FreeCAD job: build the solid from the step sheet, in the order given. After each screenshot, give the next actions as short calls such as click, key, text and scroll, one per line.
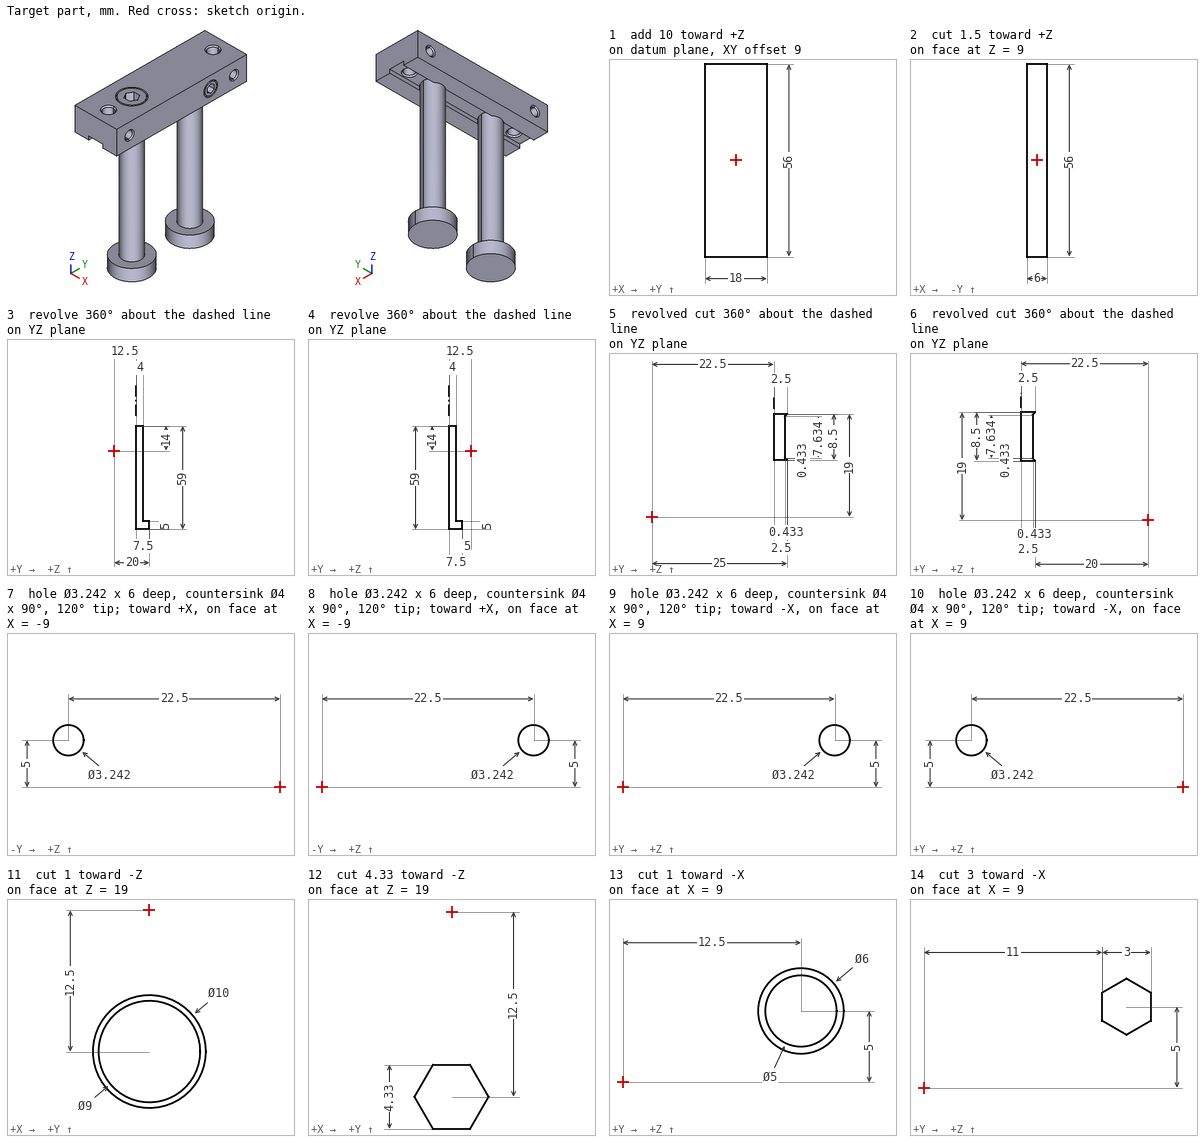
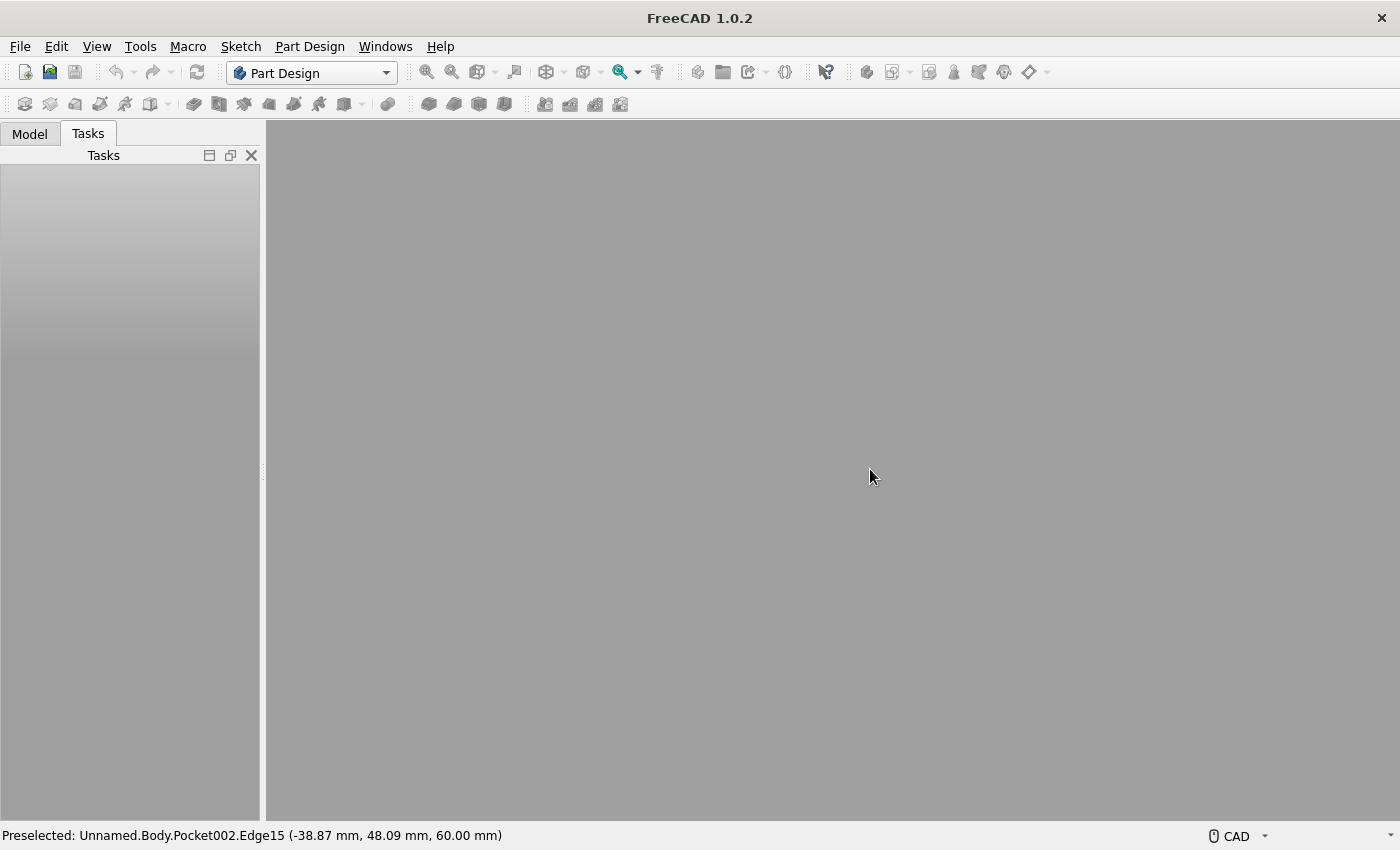
click(25, 72)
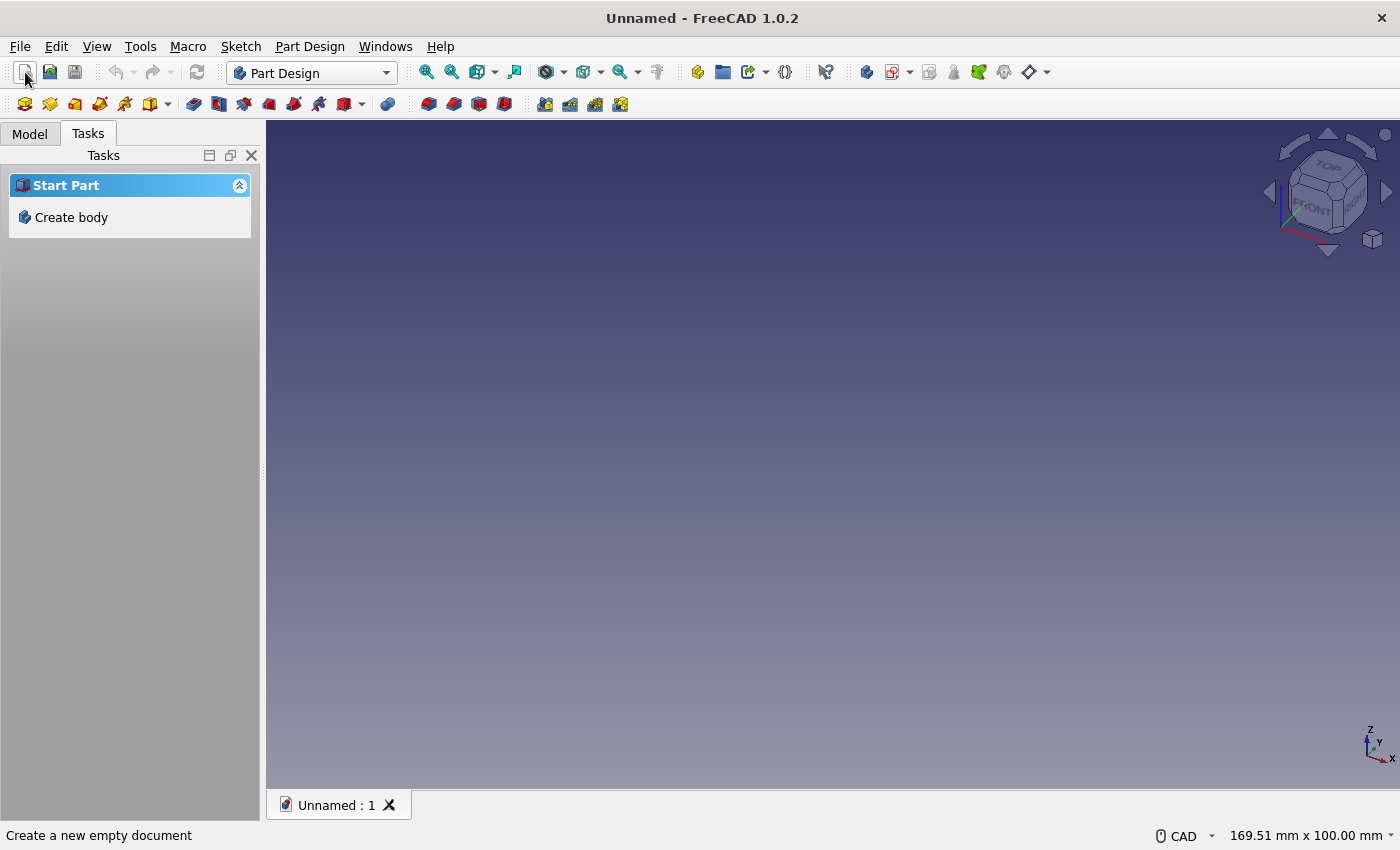
click(867, 72)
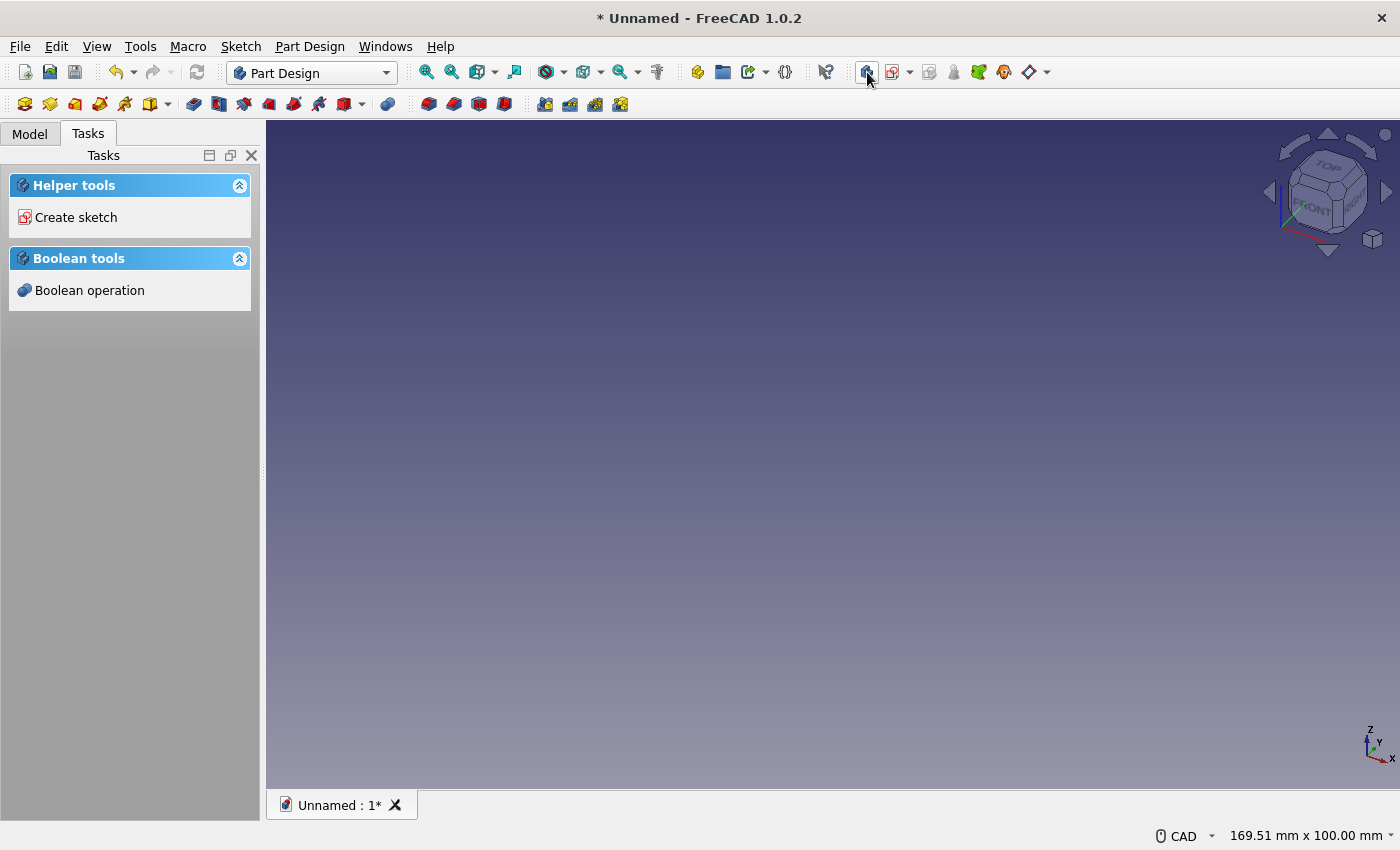
click(30, 134)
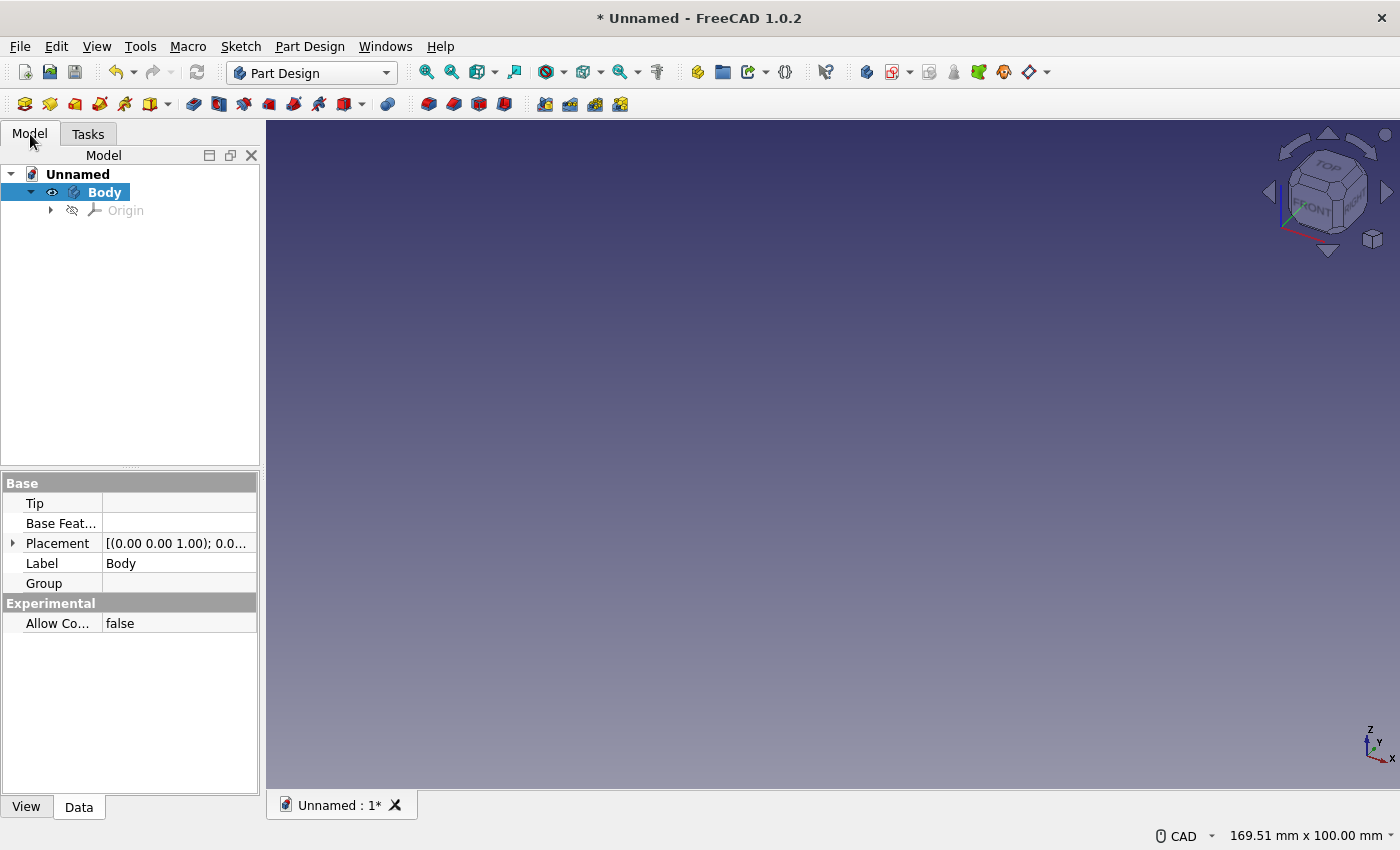
click(51, 210)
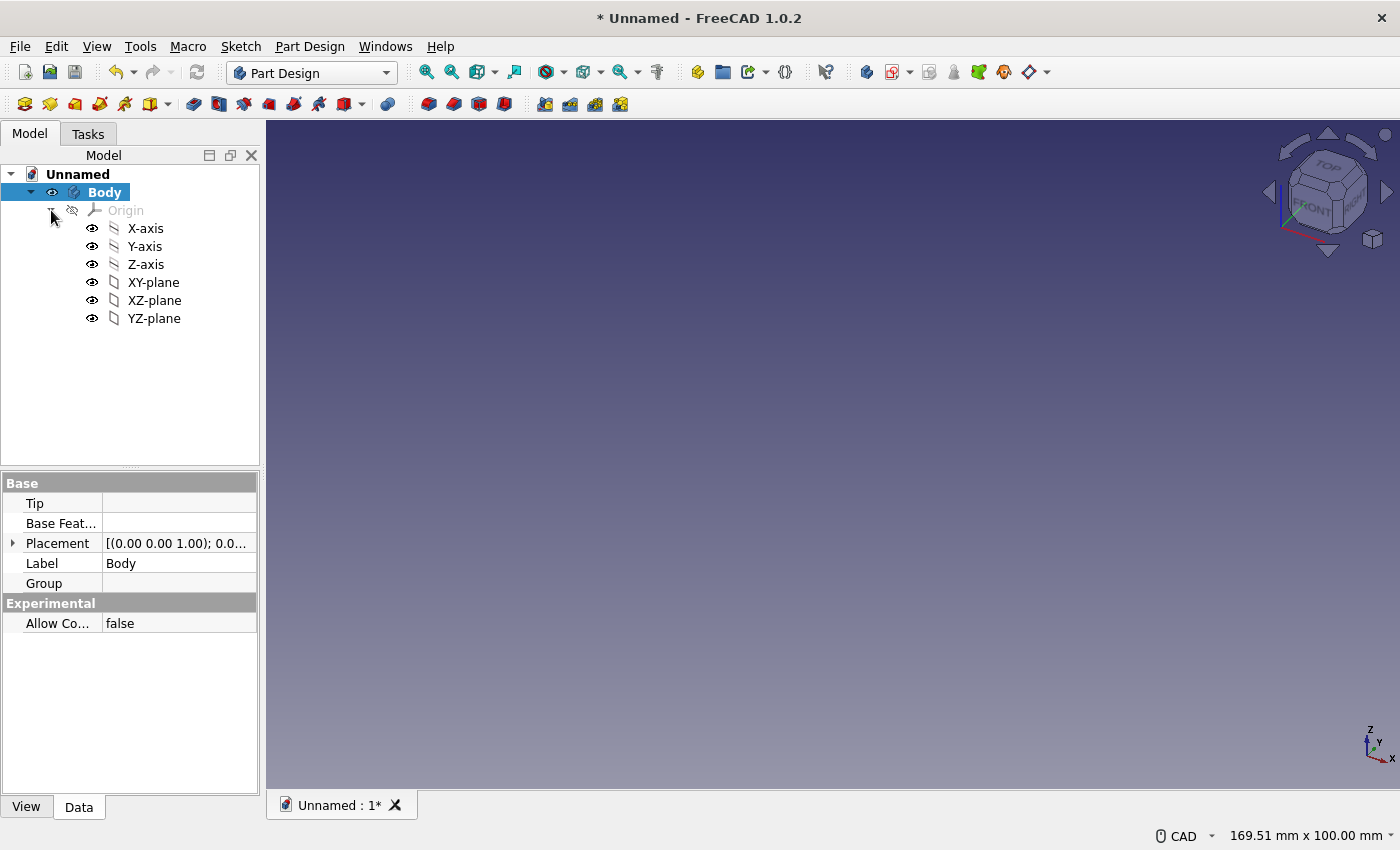
click(137, 282)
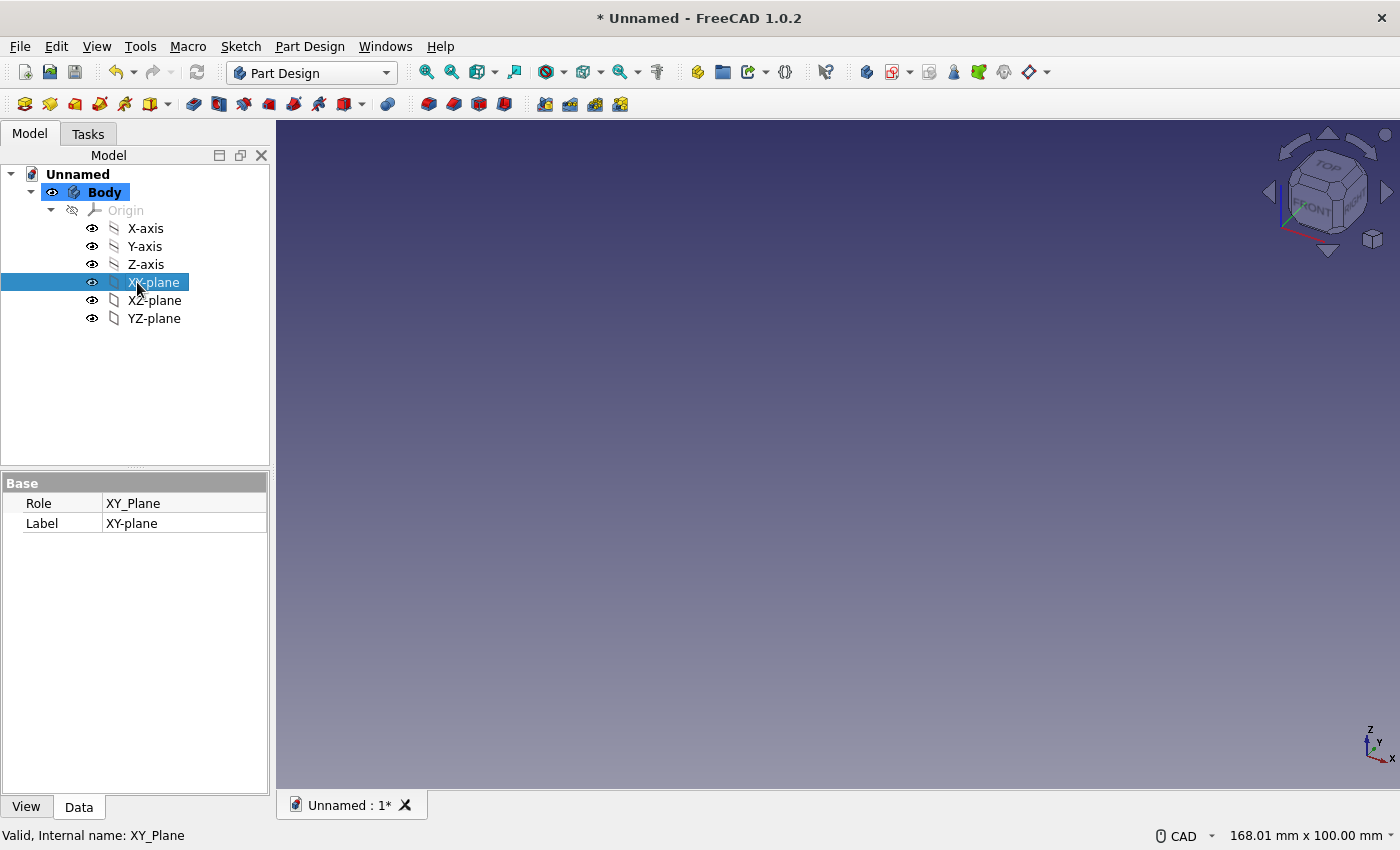
click(1028, 72)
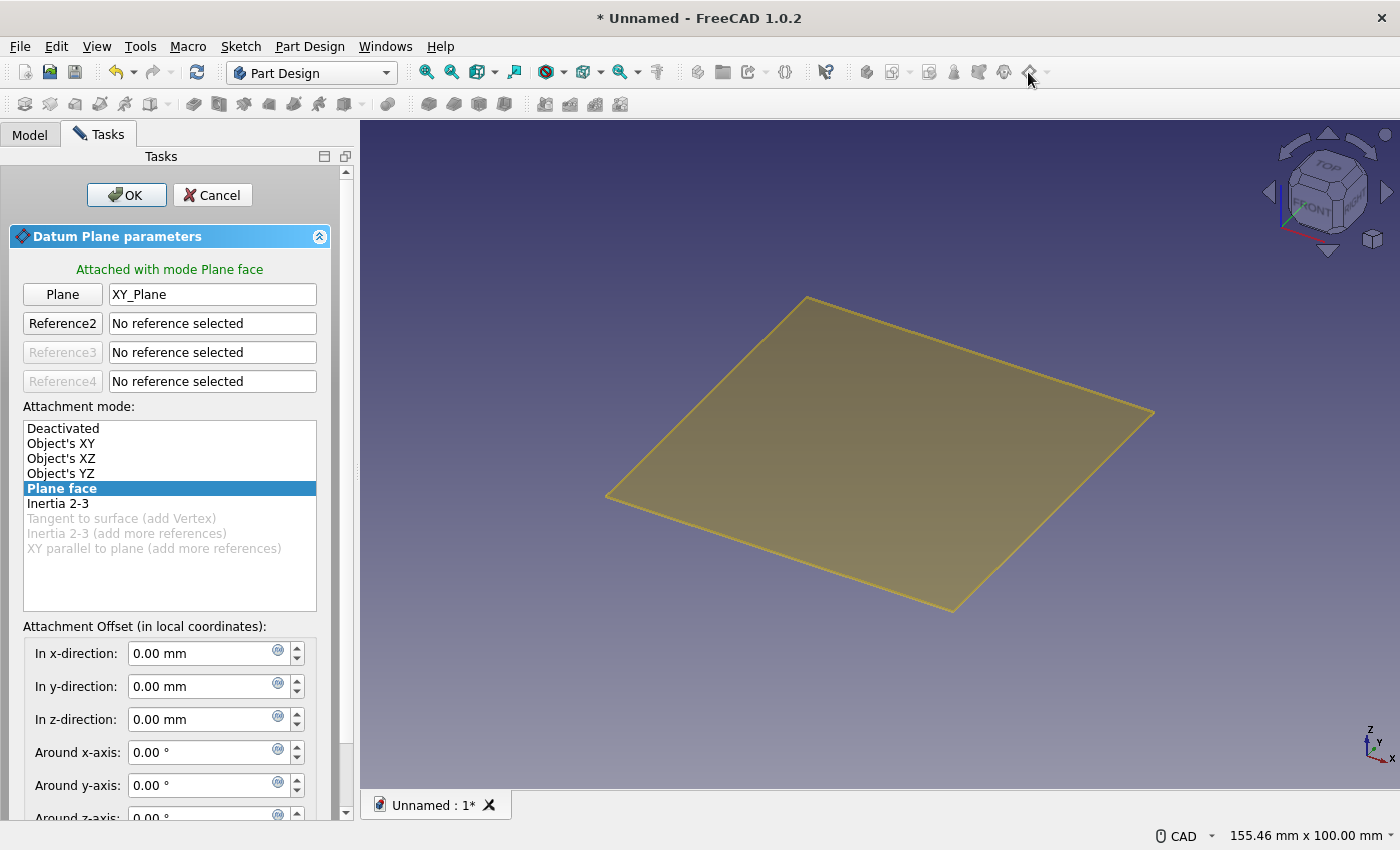
triple_click(210, 720)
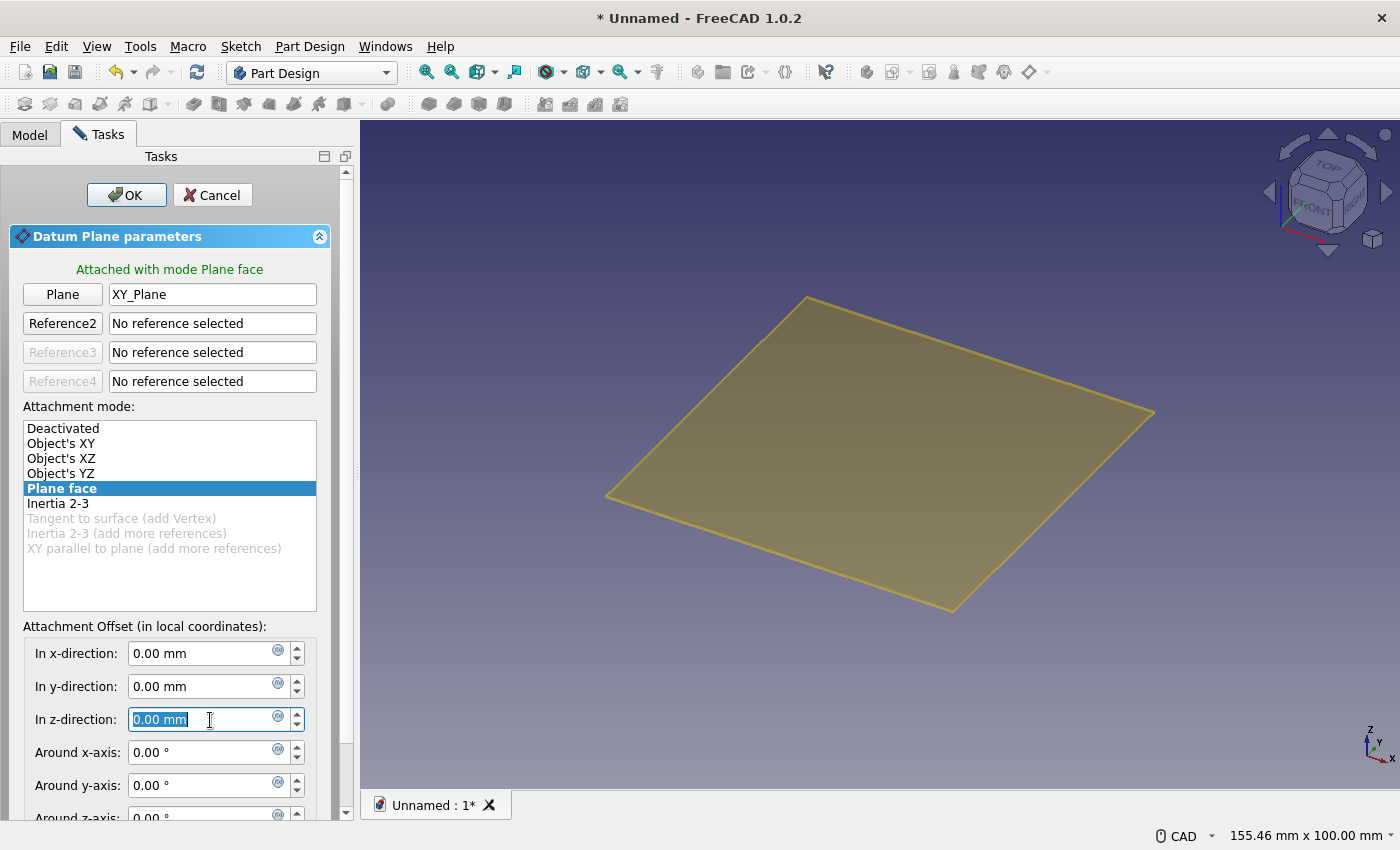
text(9)
key(Tab)